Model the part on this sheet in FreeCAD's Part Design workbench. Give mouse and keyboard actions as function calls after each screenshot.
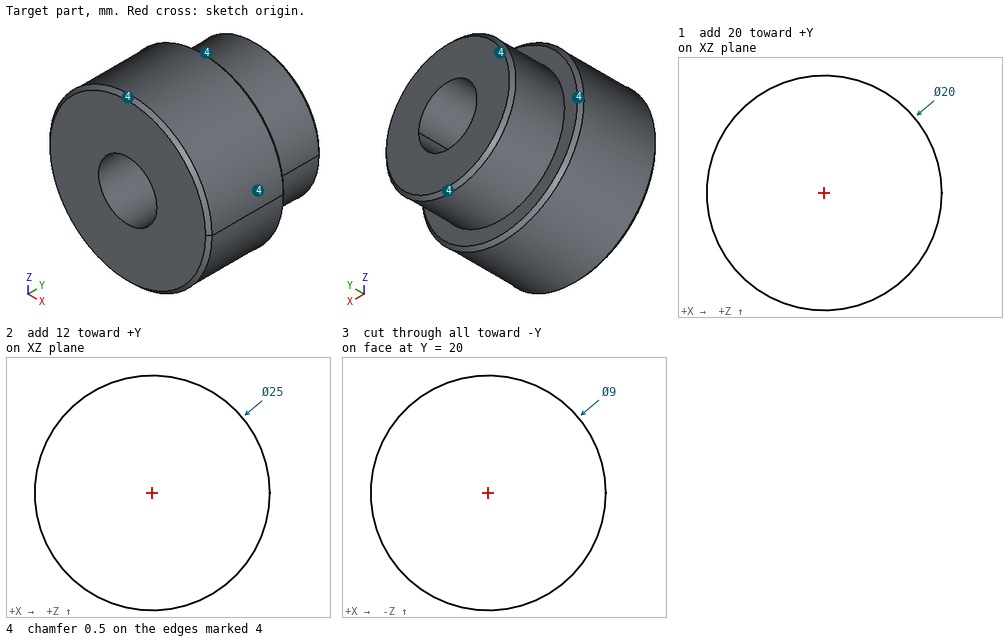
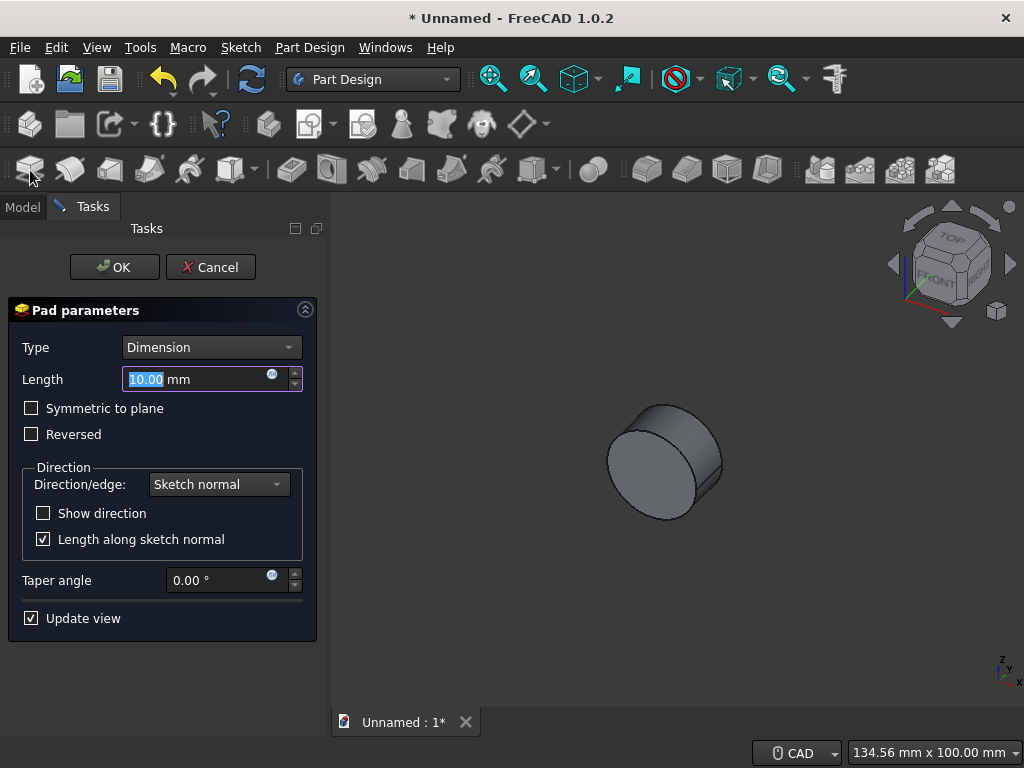
text(20)
key(Tab)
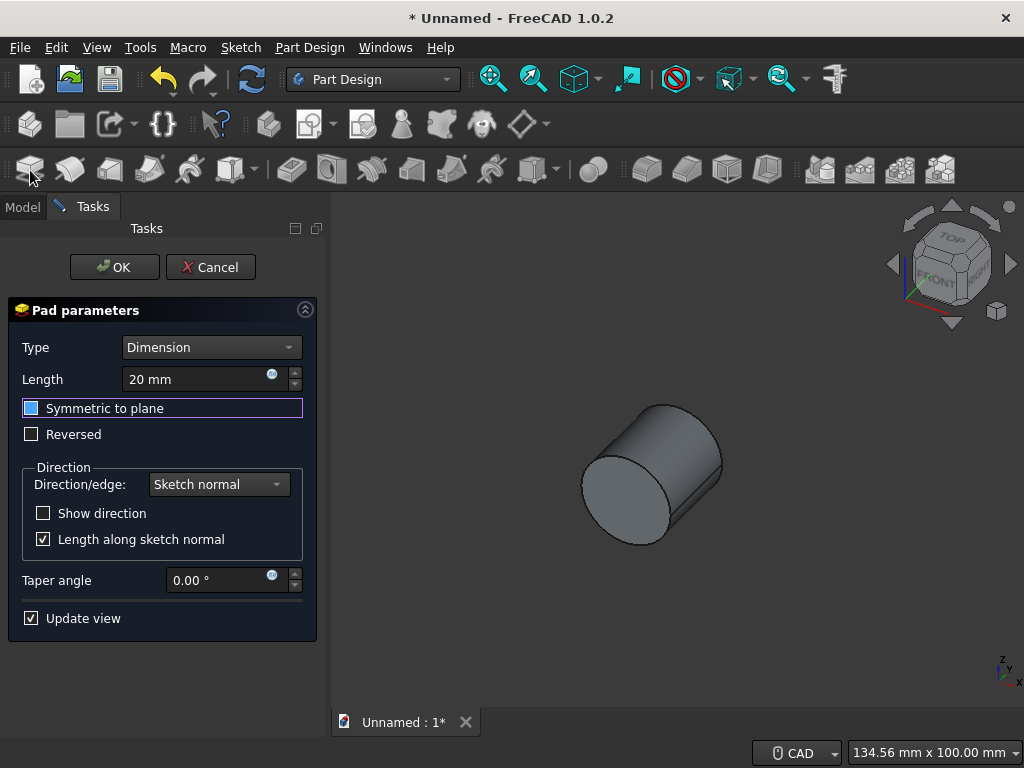
click(30, 434)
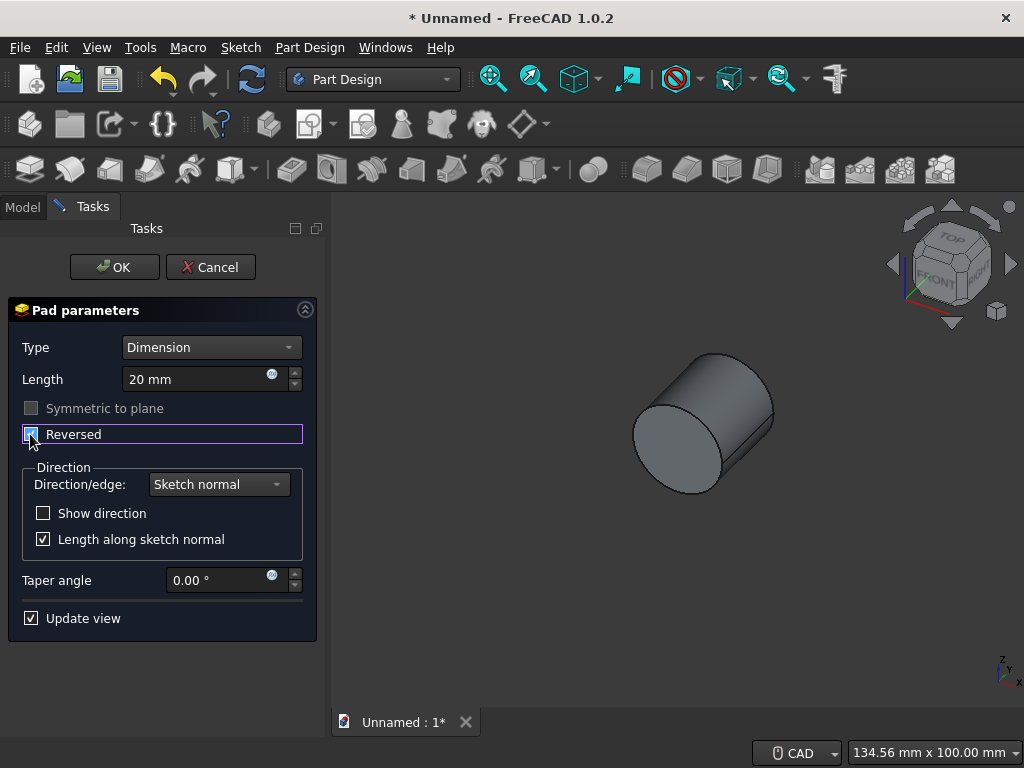
click(115, 267)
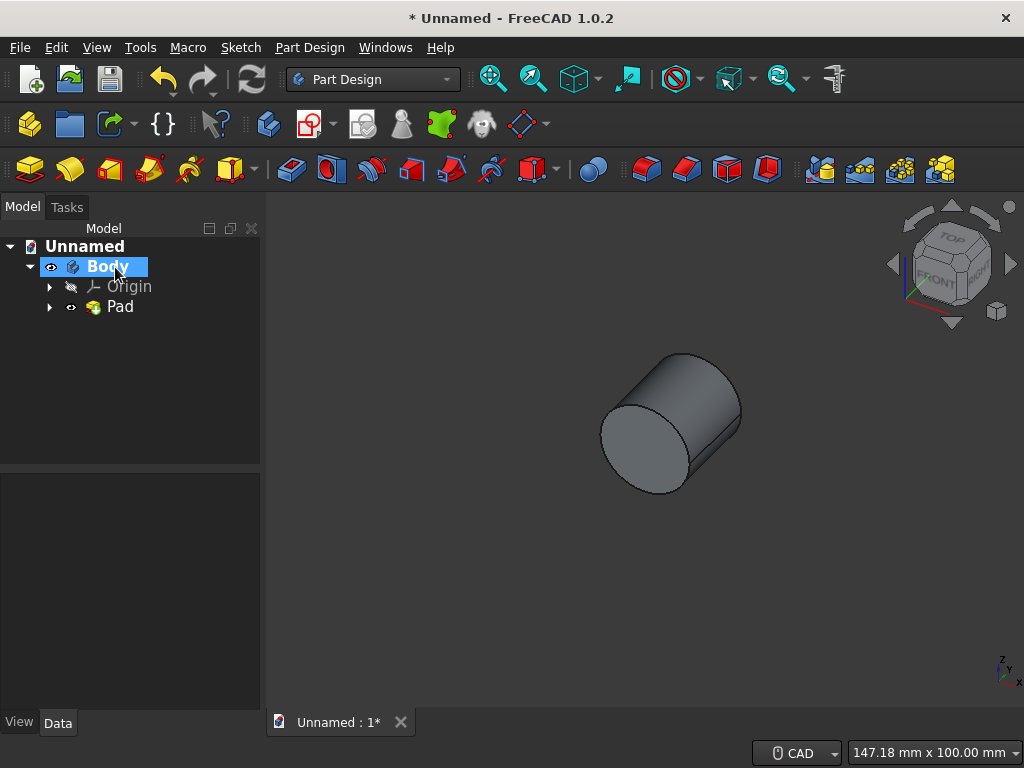
key(v)
key(f)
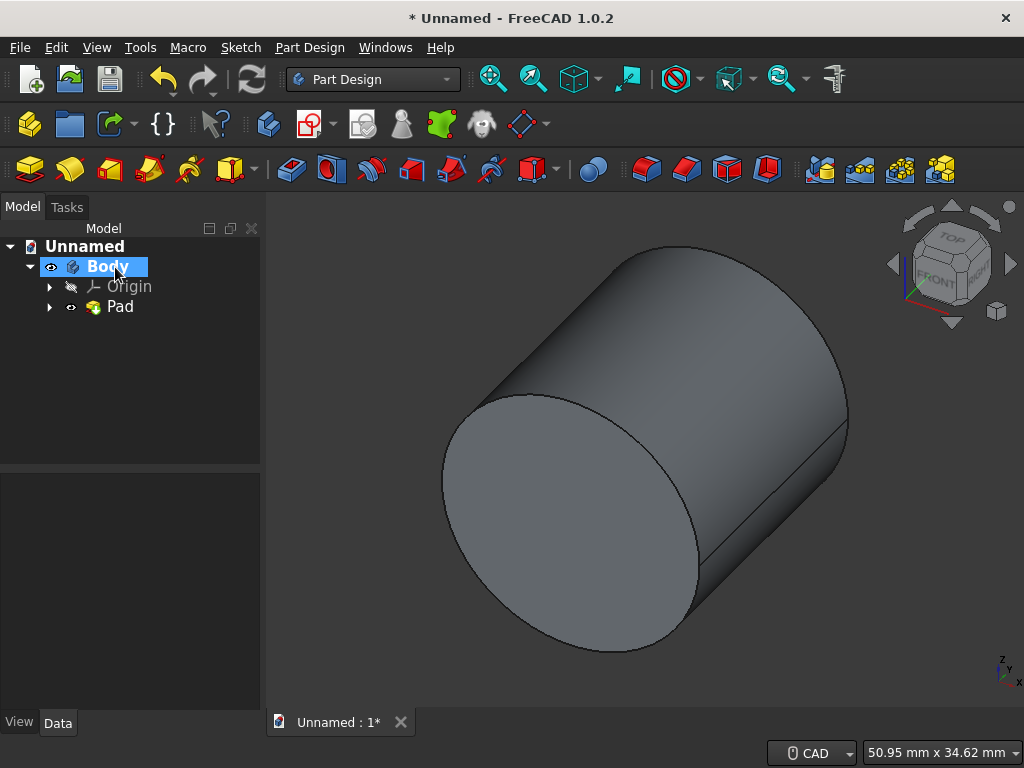
click(310, 124)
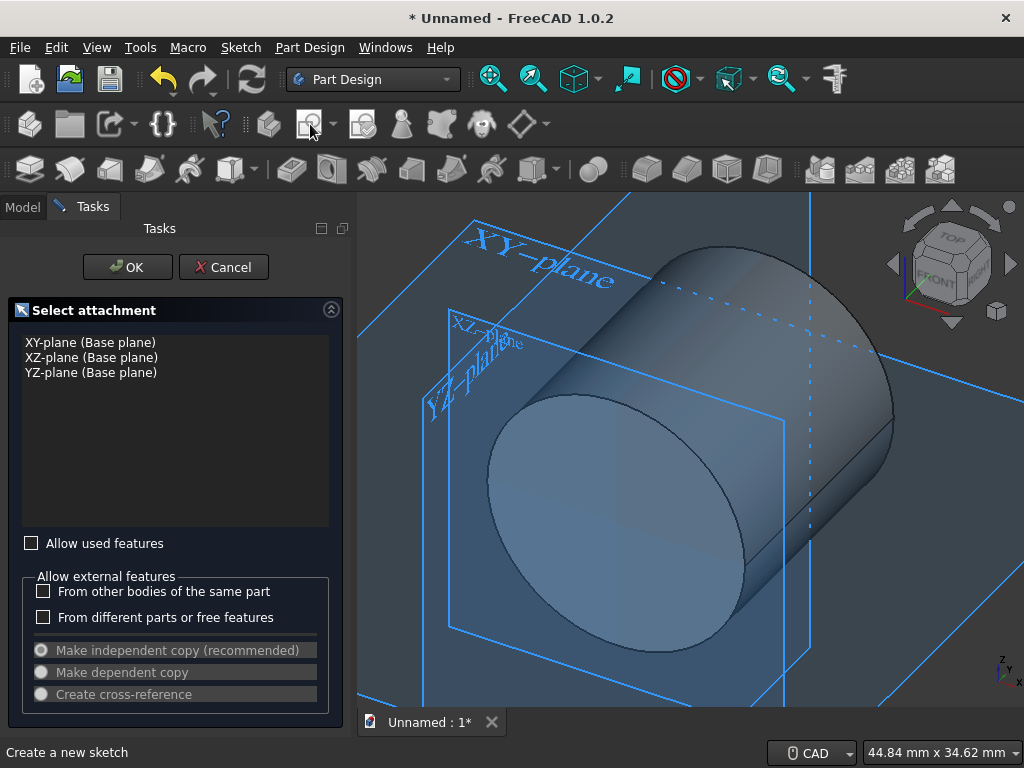
click(82, 358)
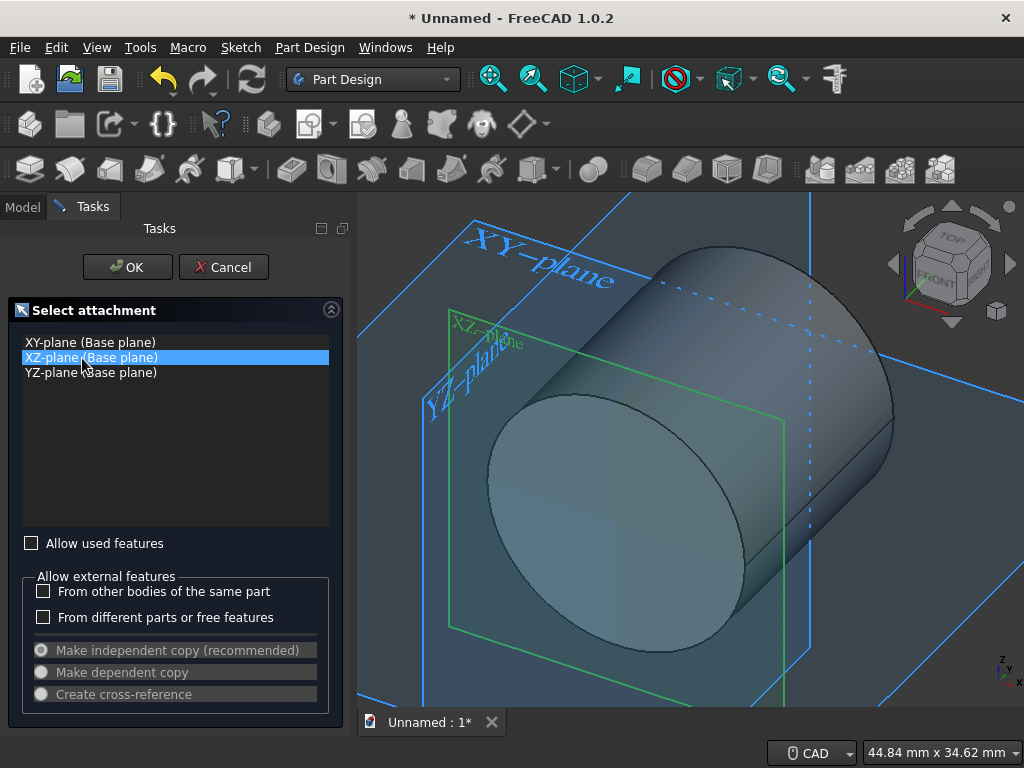
click(128, 267)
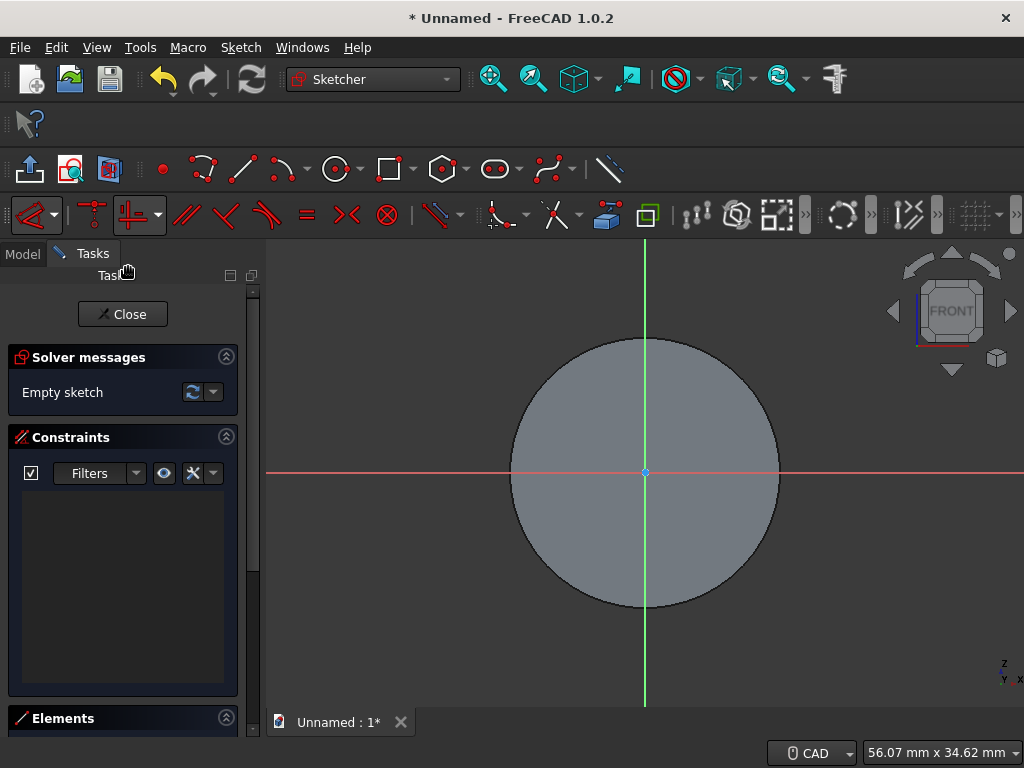
click(336, 170)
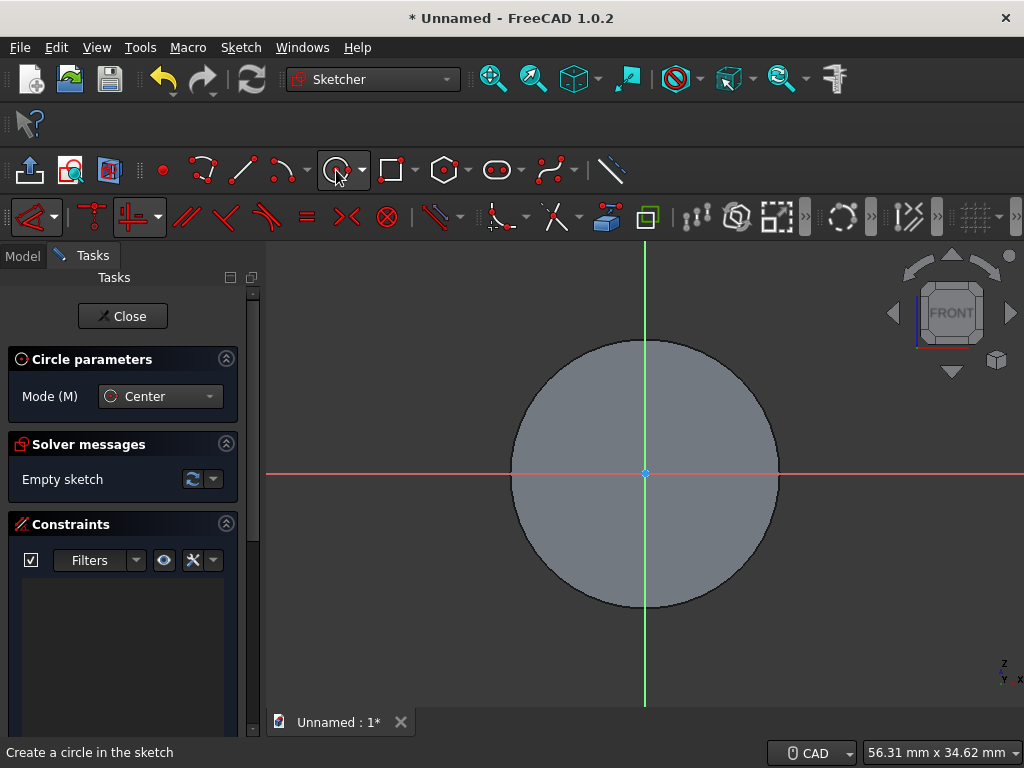
click(645, 474)
click(764, 355)
key(Escape)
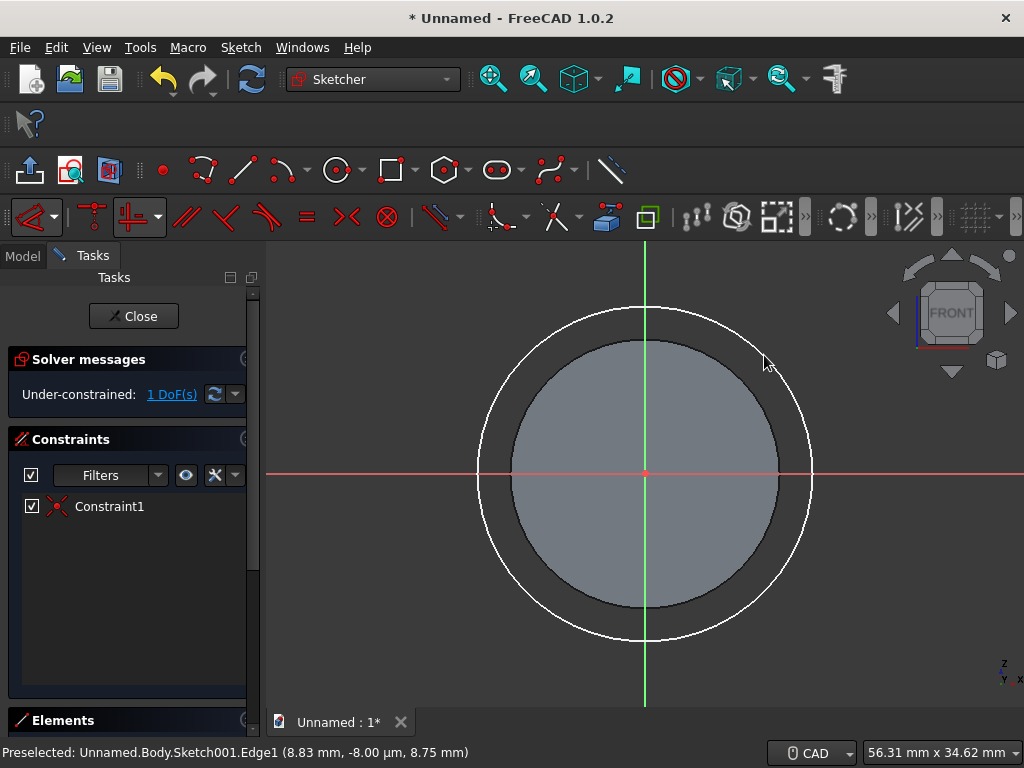
click(763, 355)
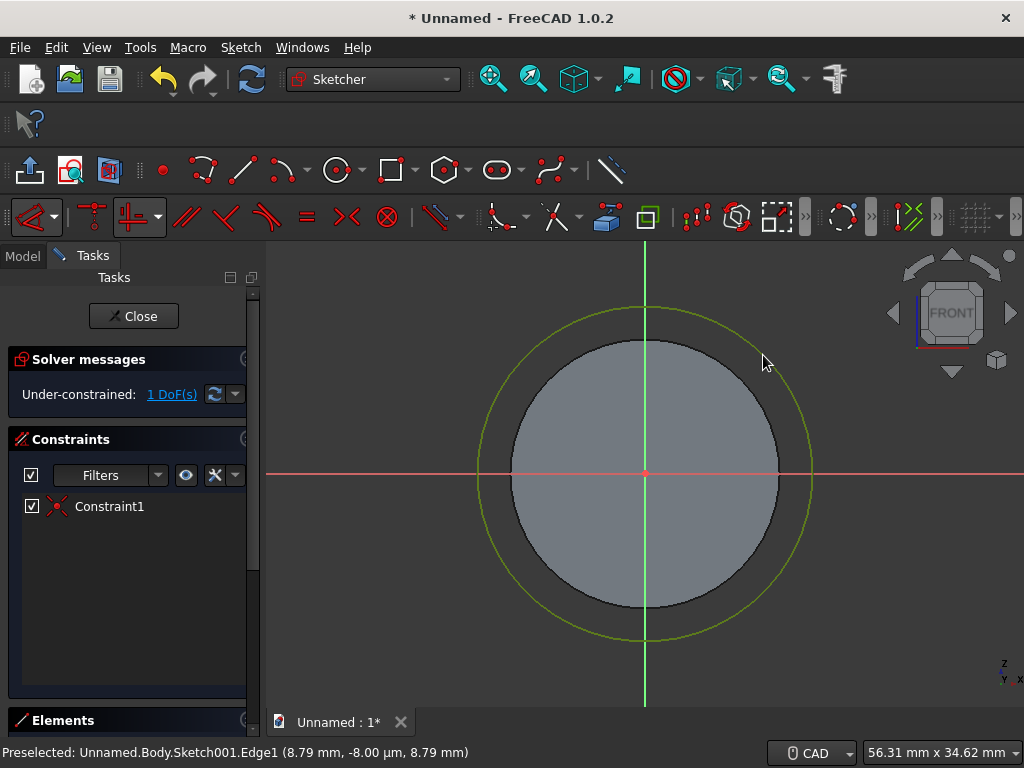
key(k)
key(o)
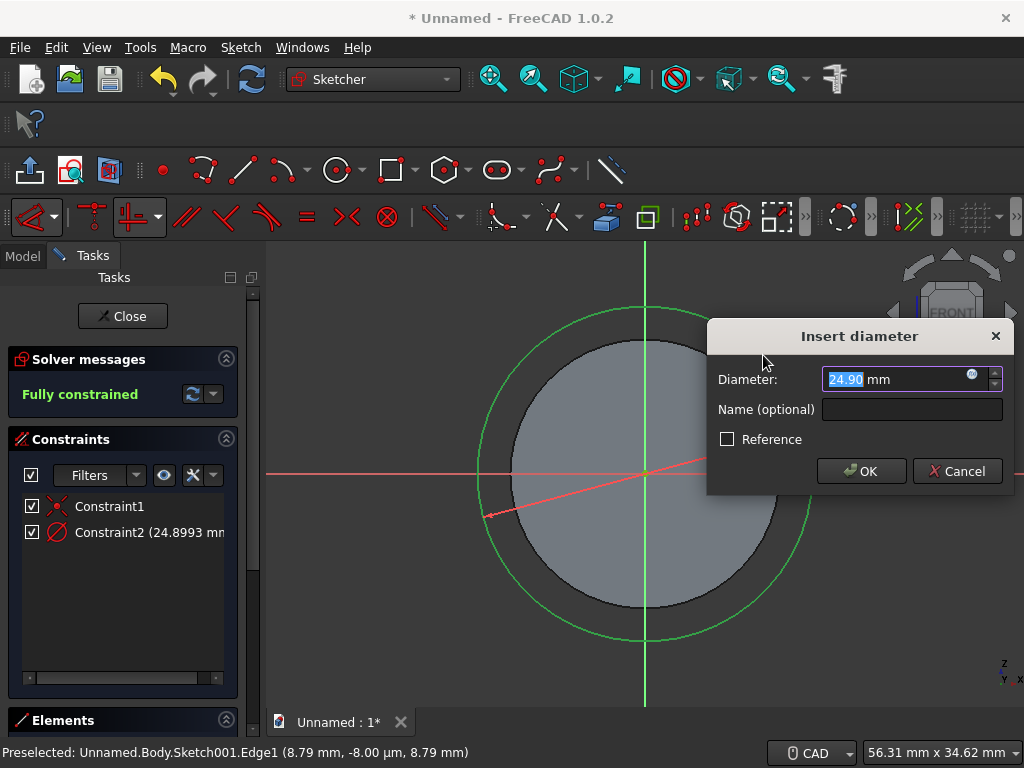
text(25)
key(Return)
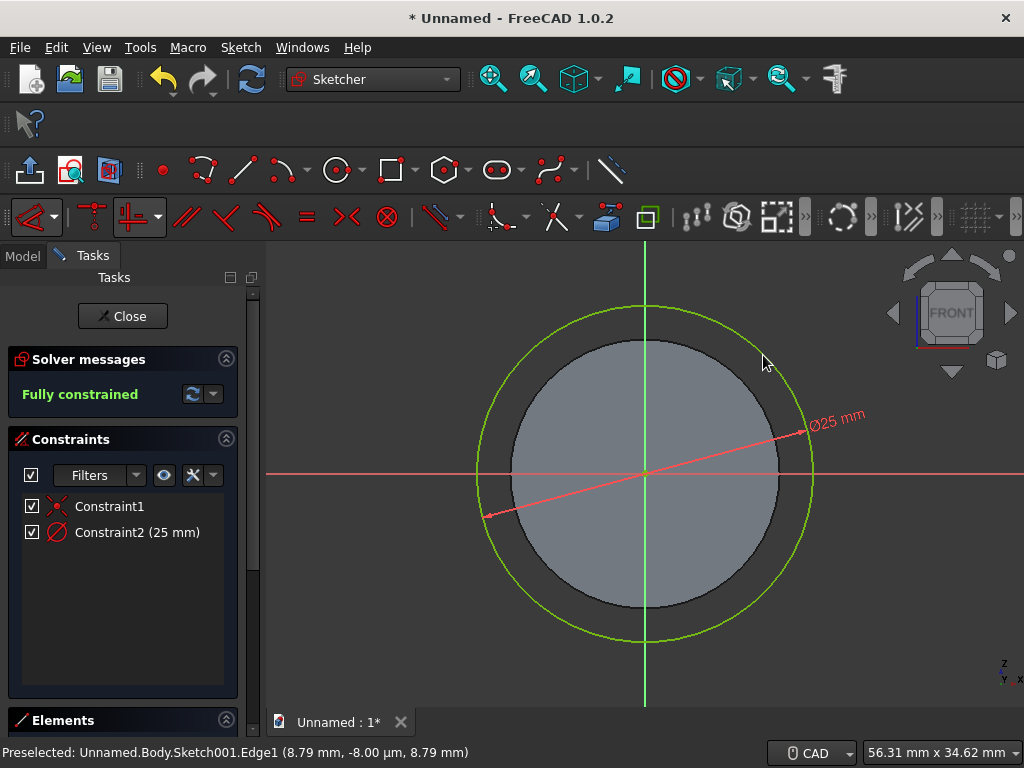
click(123, 316)